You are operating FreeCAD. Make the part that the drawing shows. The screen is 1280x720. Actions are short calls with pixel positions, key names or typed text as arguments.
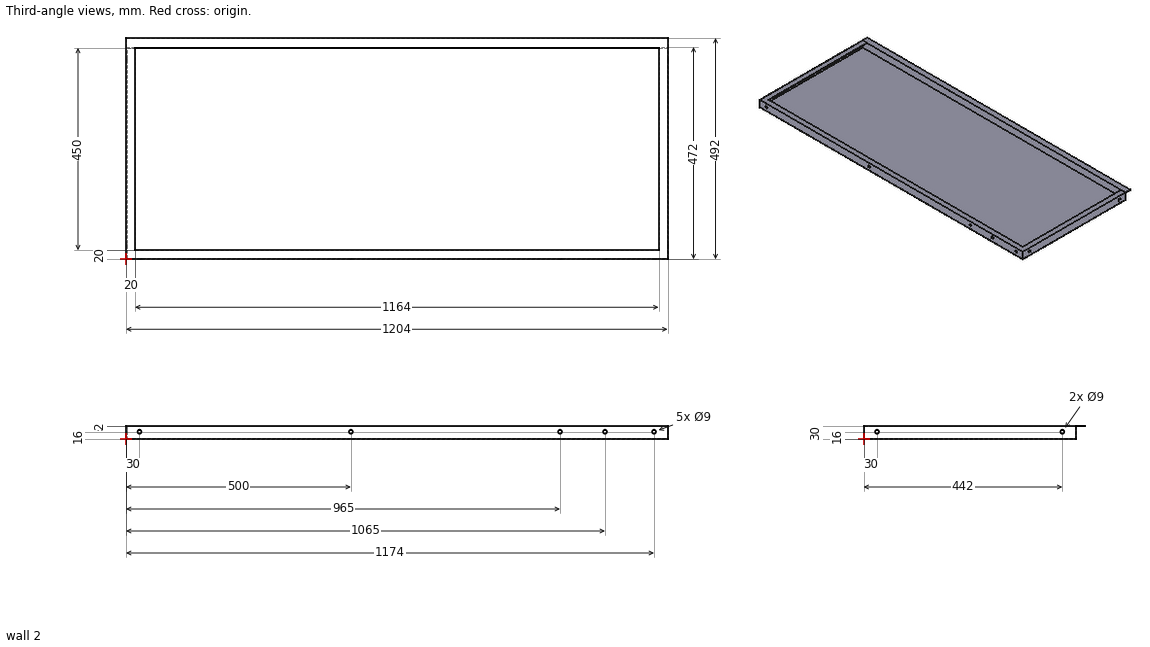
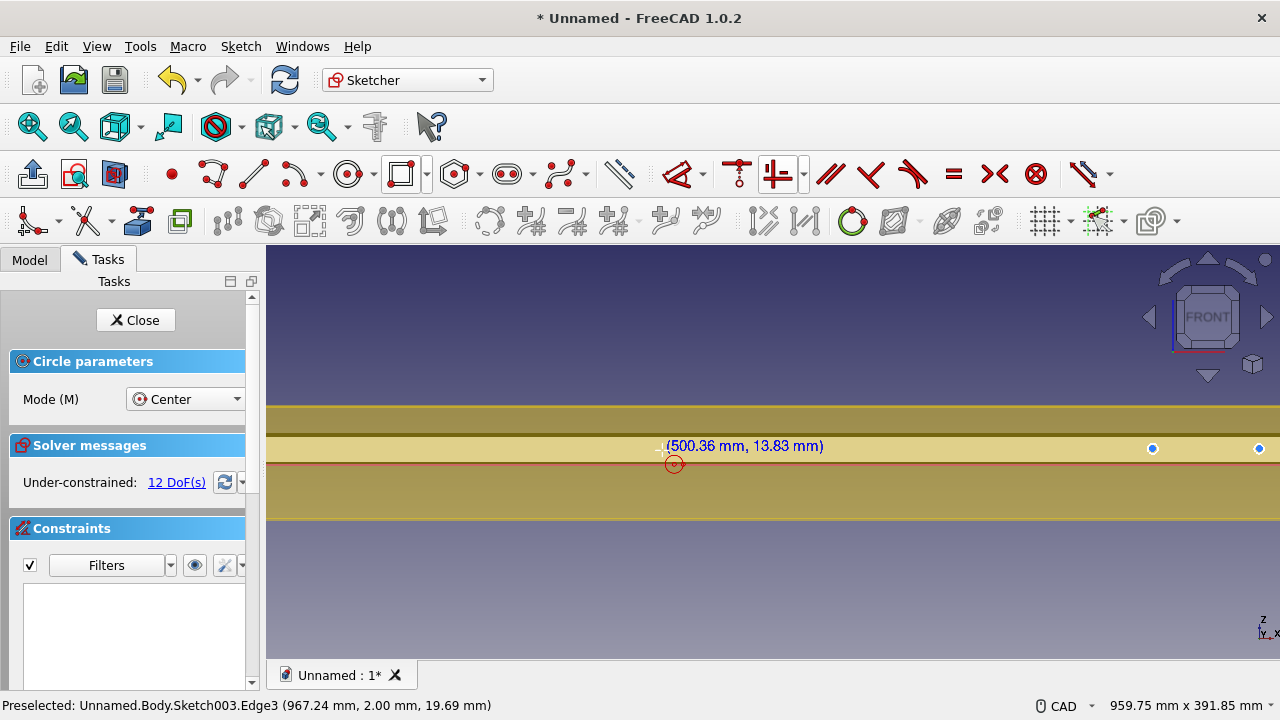
click(662, 448)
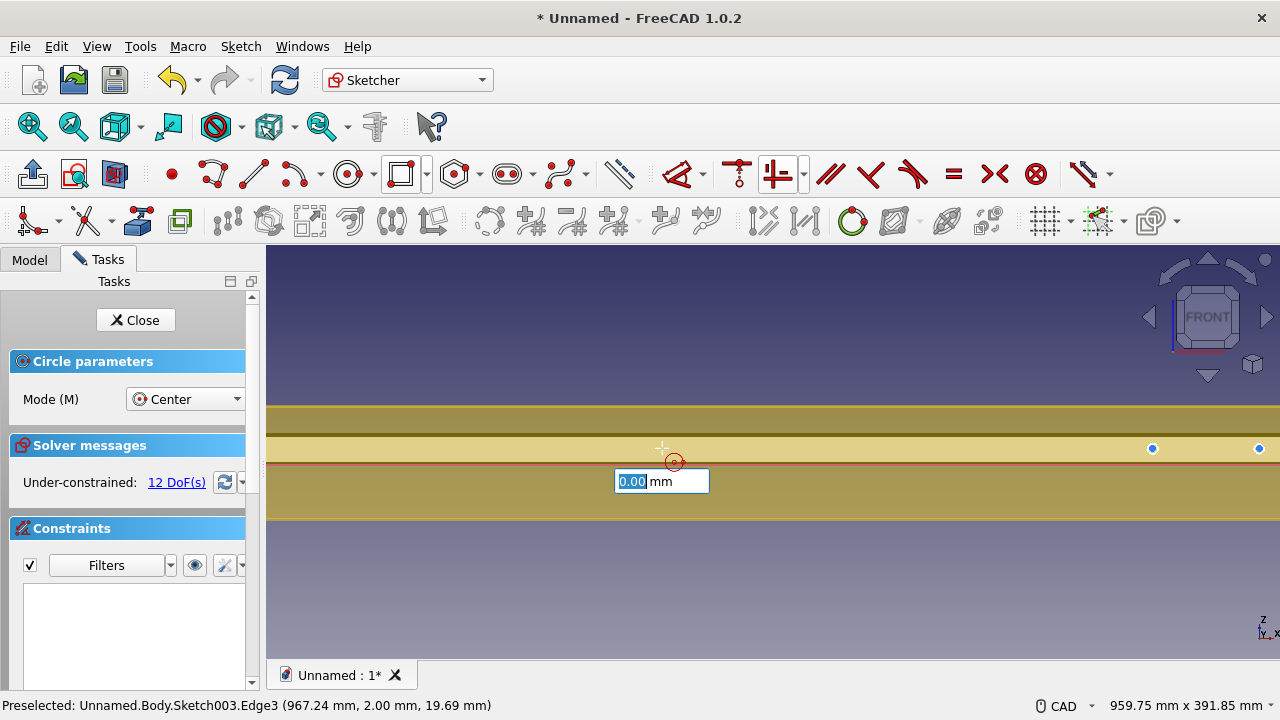
scroll(665, 445, up, 7)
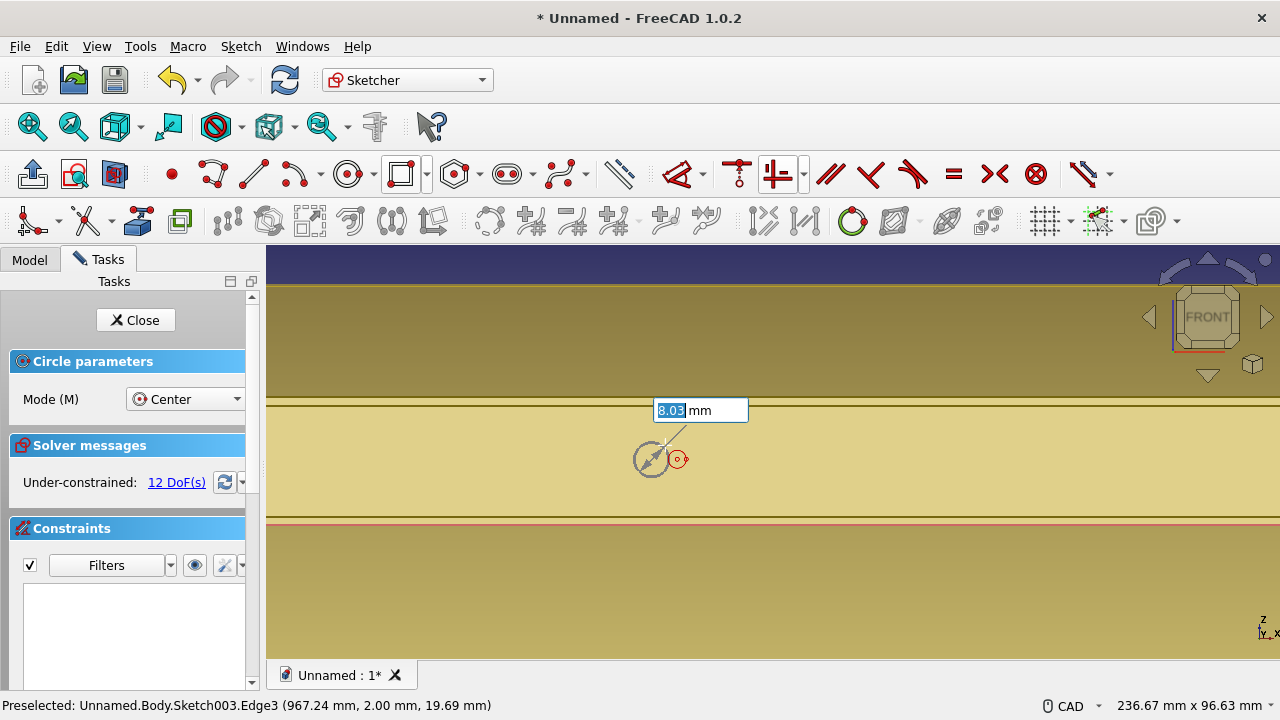
click(665, 443)
key(Escape)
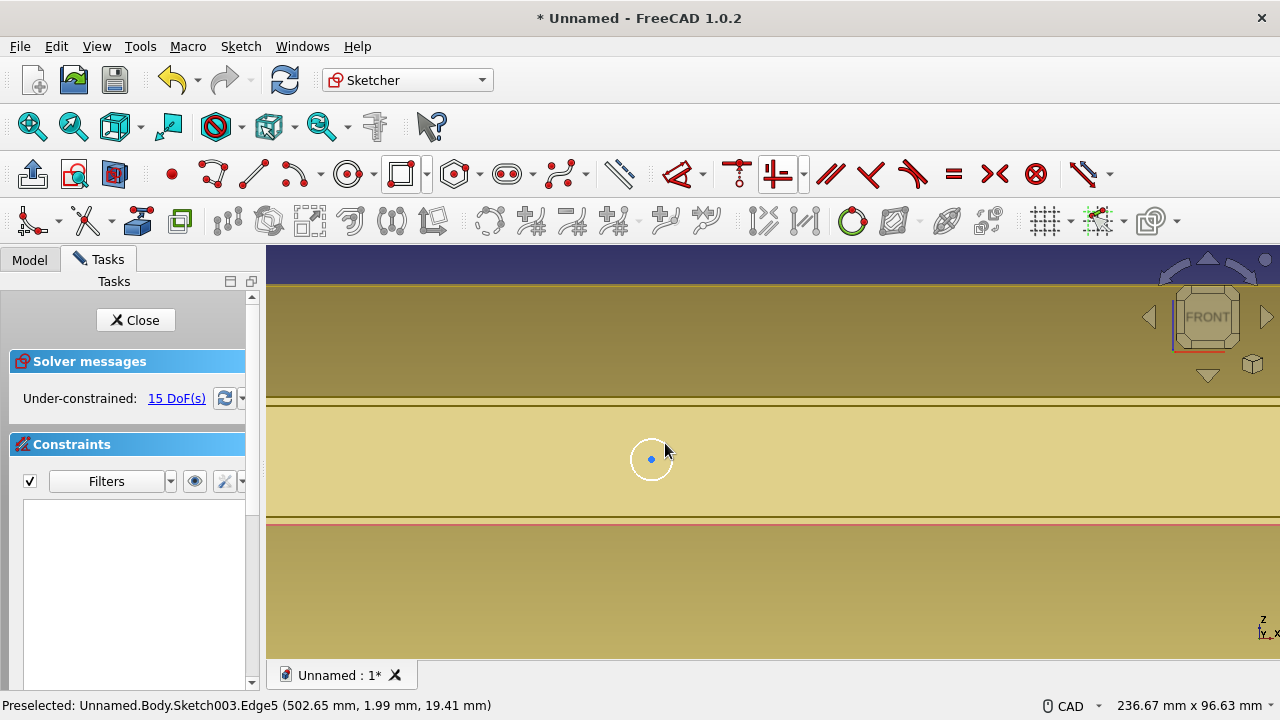
scroll(663, 448, down, 11)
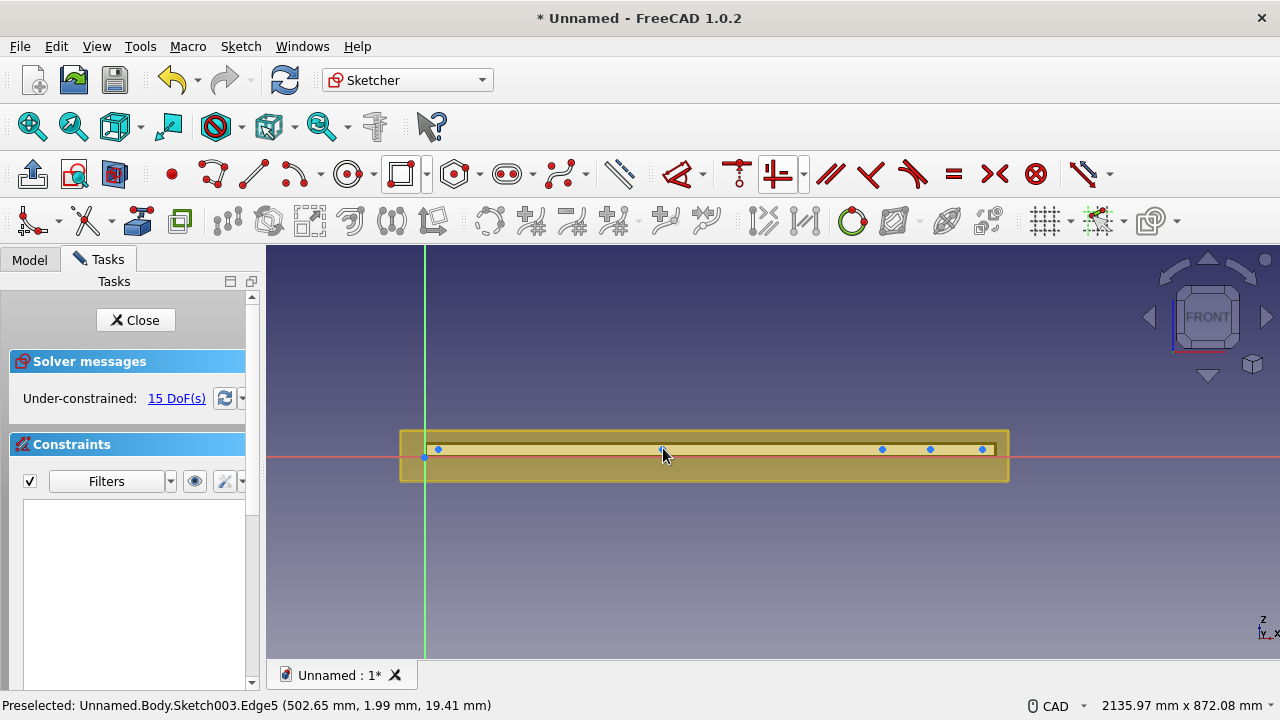
scroll(984, 448, up, 9)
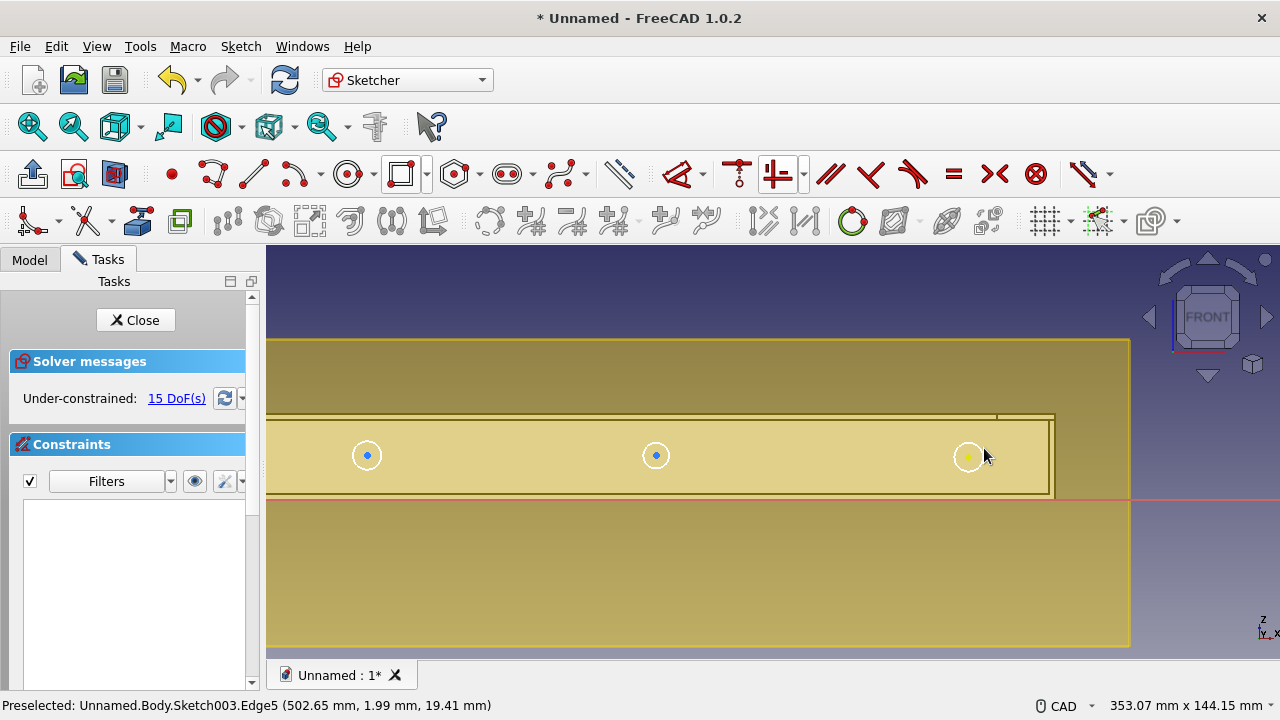
click(979, 447)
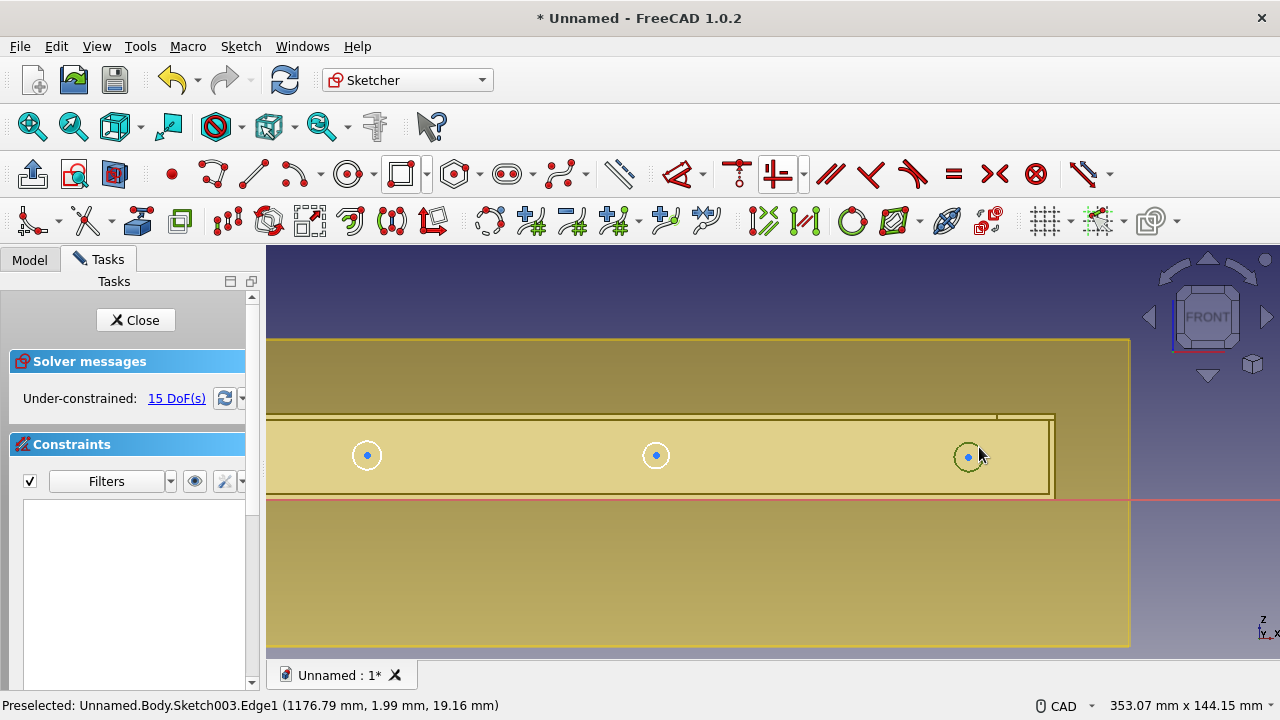
scroll(985, 448, down, 9)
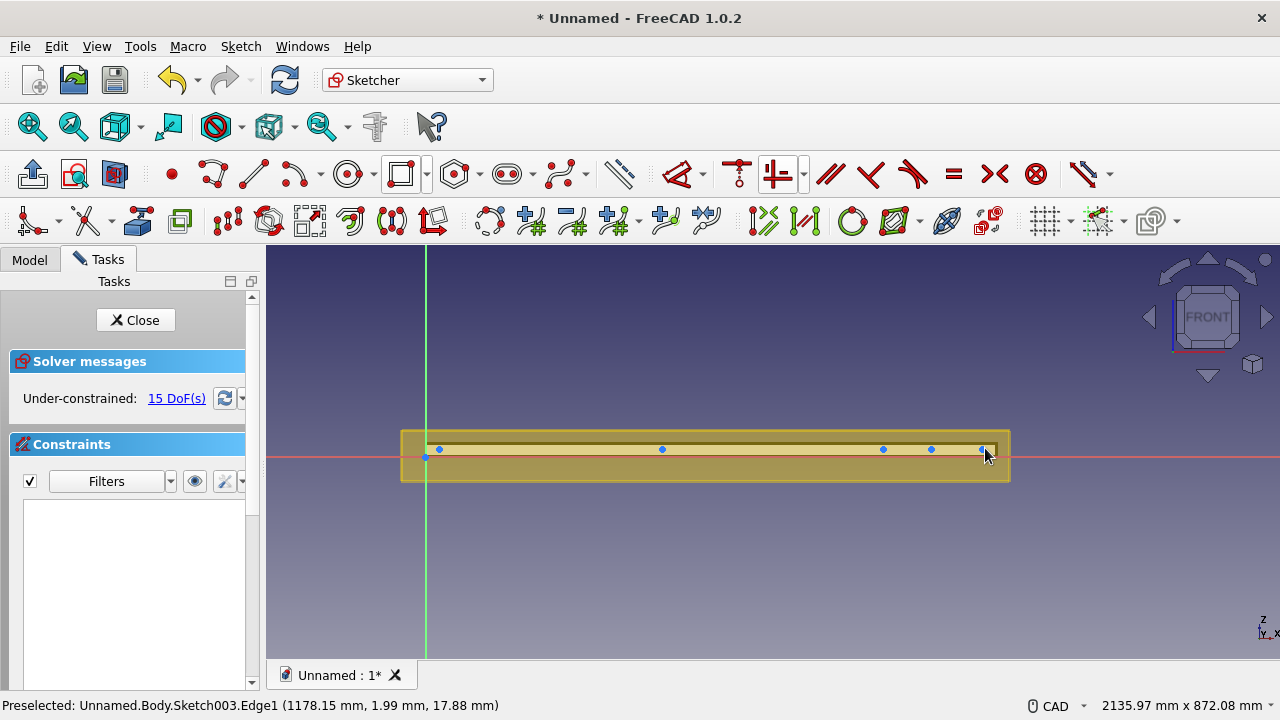
scroll(441, 448, up, 9)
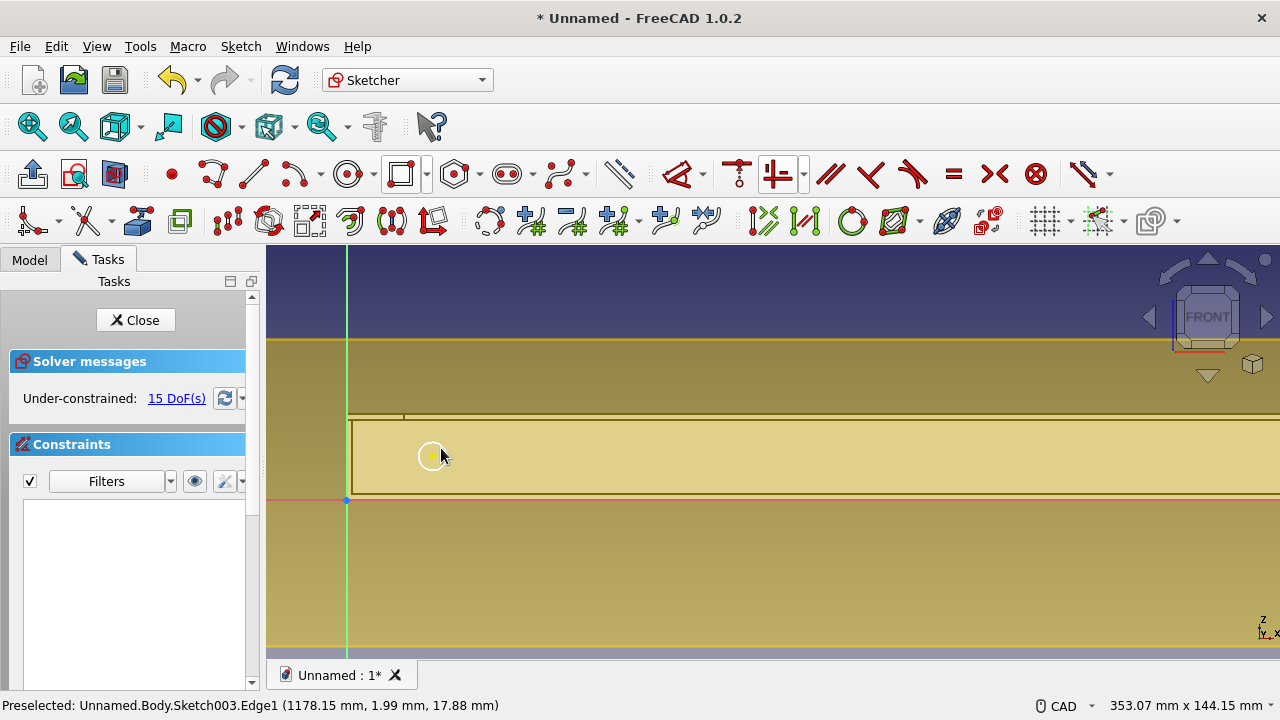
click(443, 447)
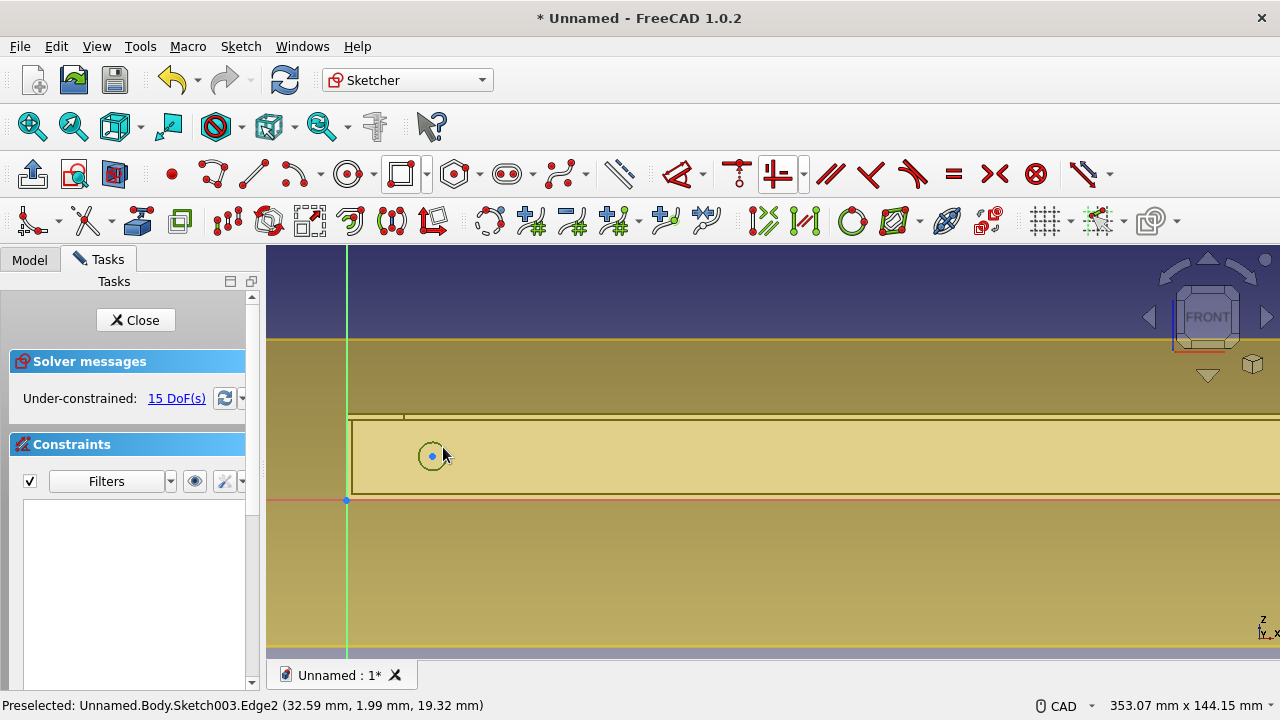
scroll(440, 448, down, 9)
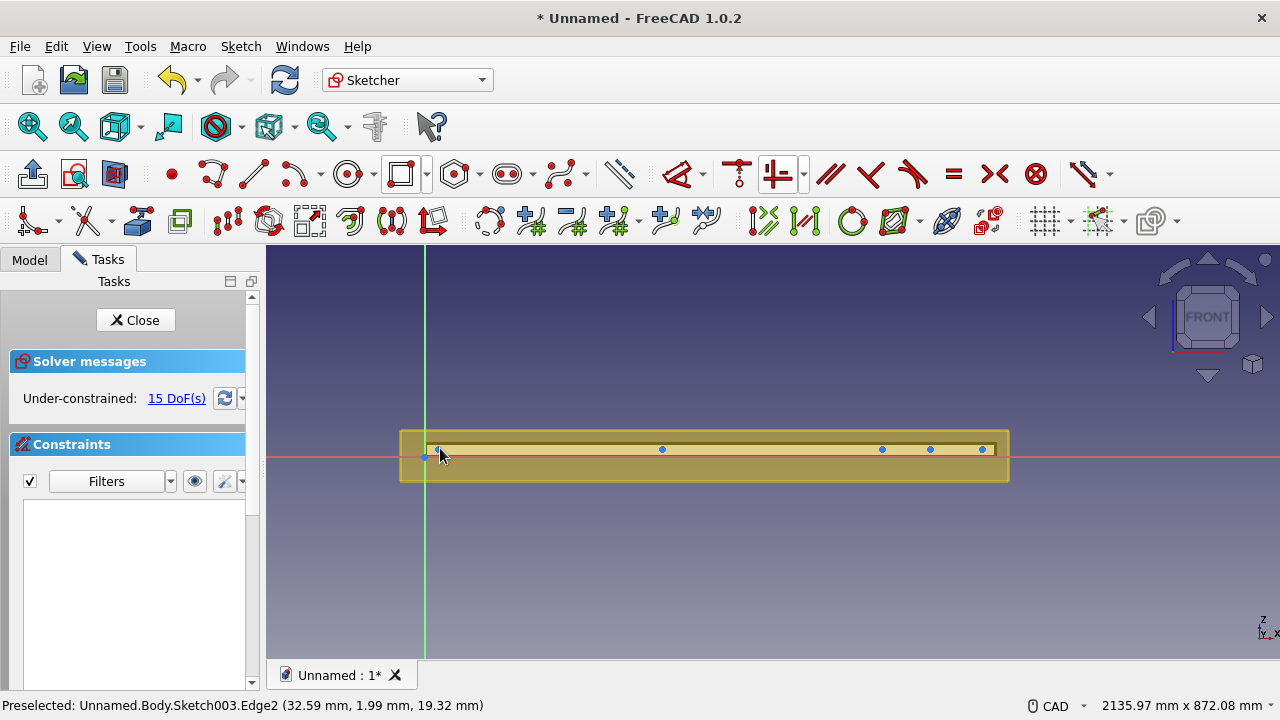
scroll(932, 448, up, 10)